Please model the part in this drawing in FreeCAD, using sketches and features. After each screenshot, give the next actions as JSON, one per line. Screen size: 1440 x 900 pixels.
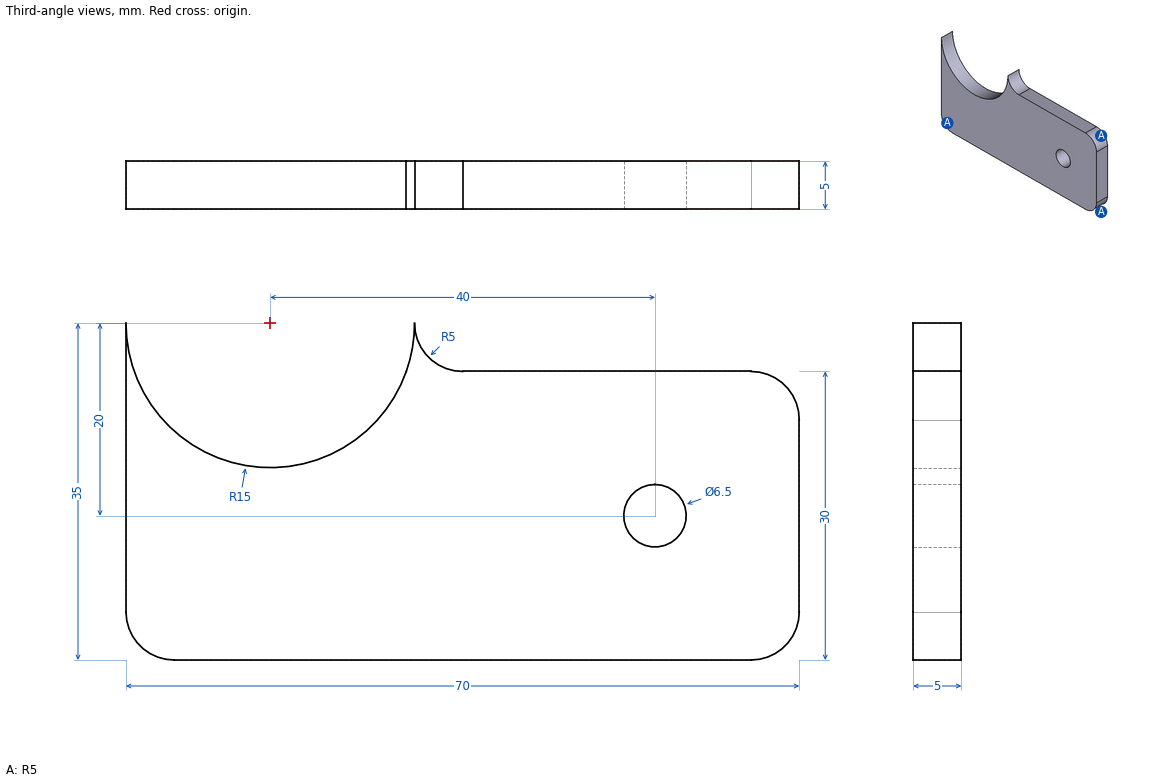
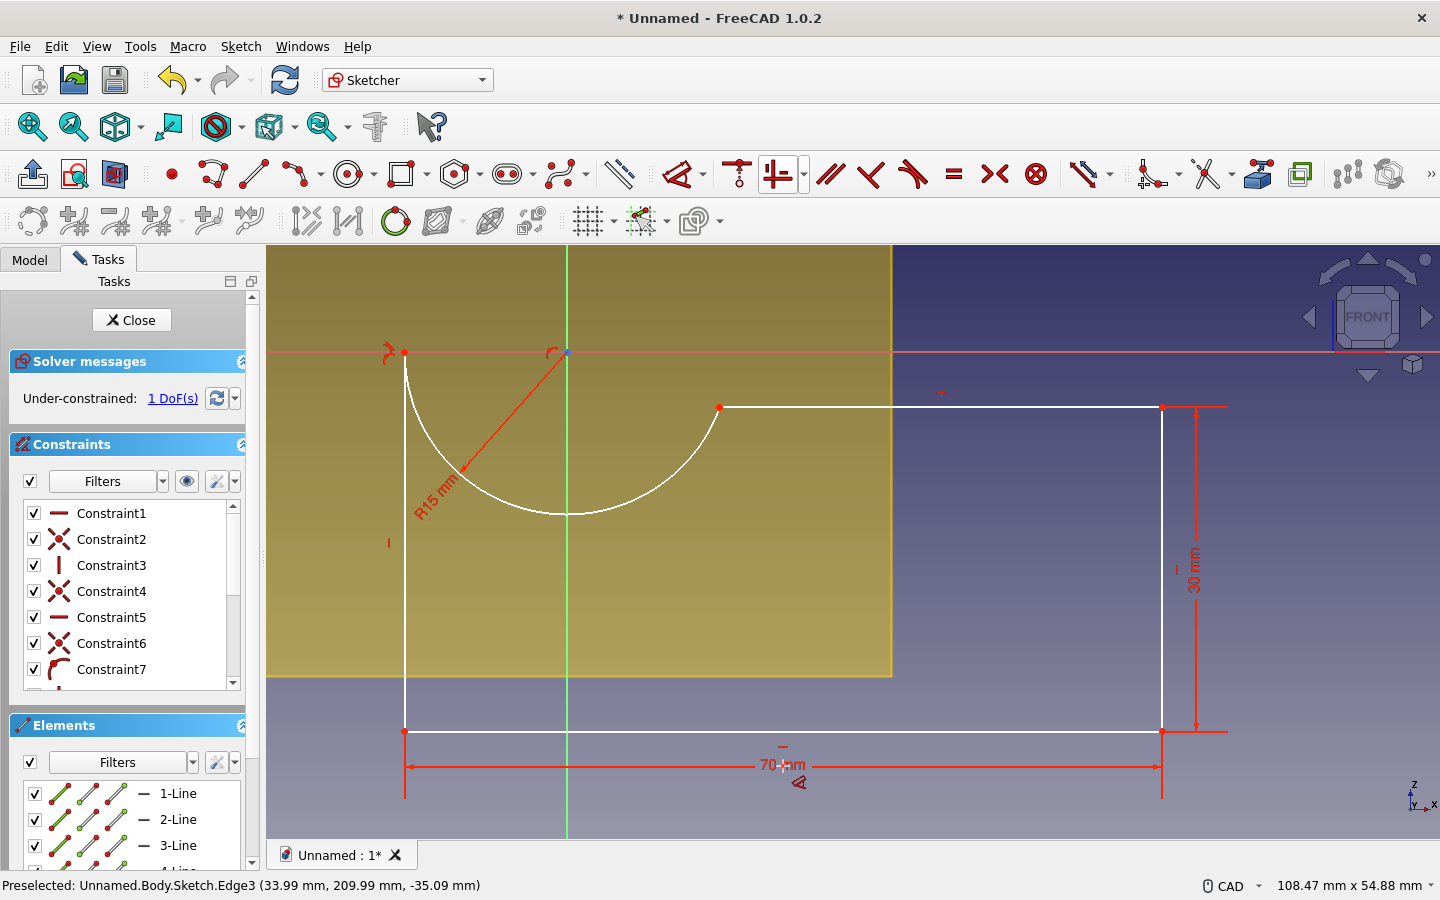
{"action": "left_click", "coordinate": [405, 618]}
{"action": "left_click", "coordinate": [371, 542]}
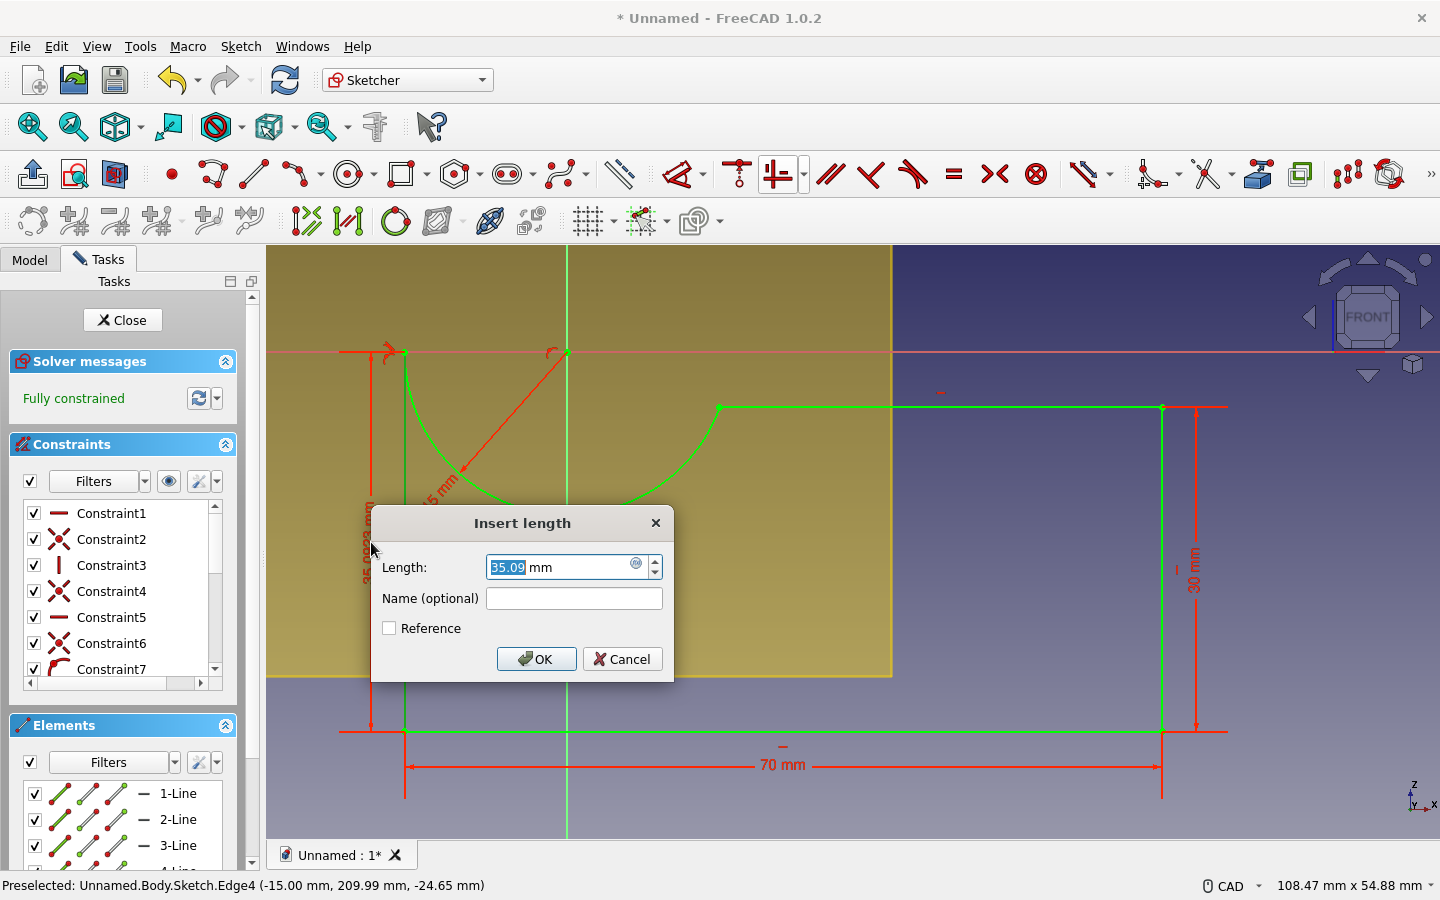
{"action": "type", "text": "35"}
{"action": "key", "text": "Return"}
{"action": "key", "text": "Escape"}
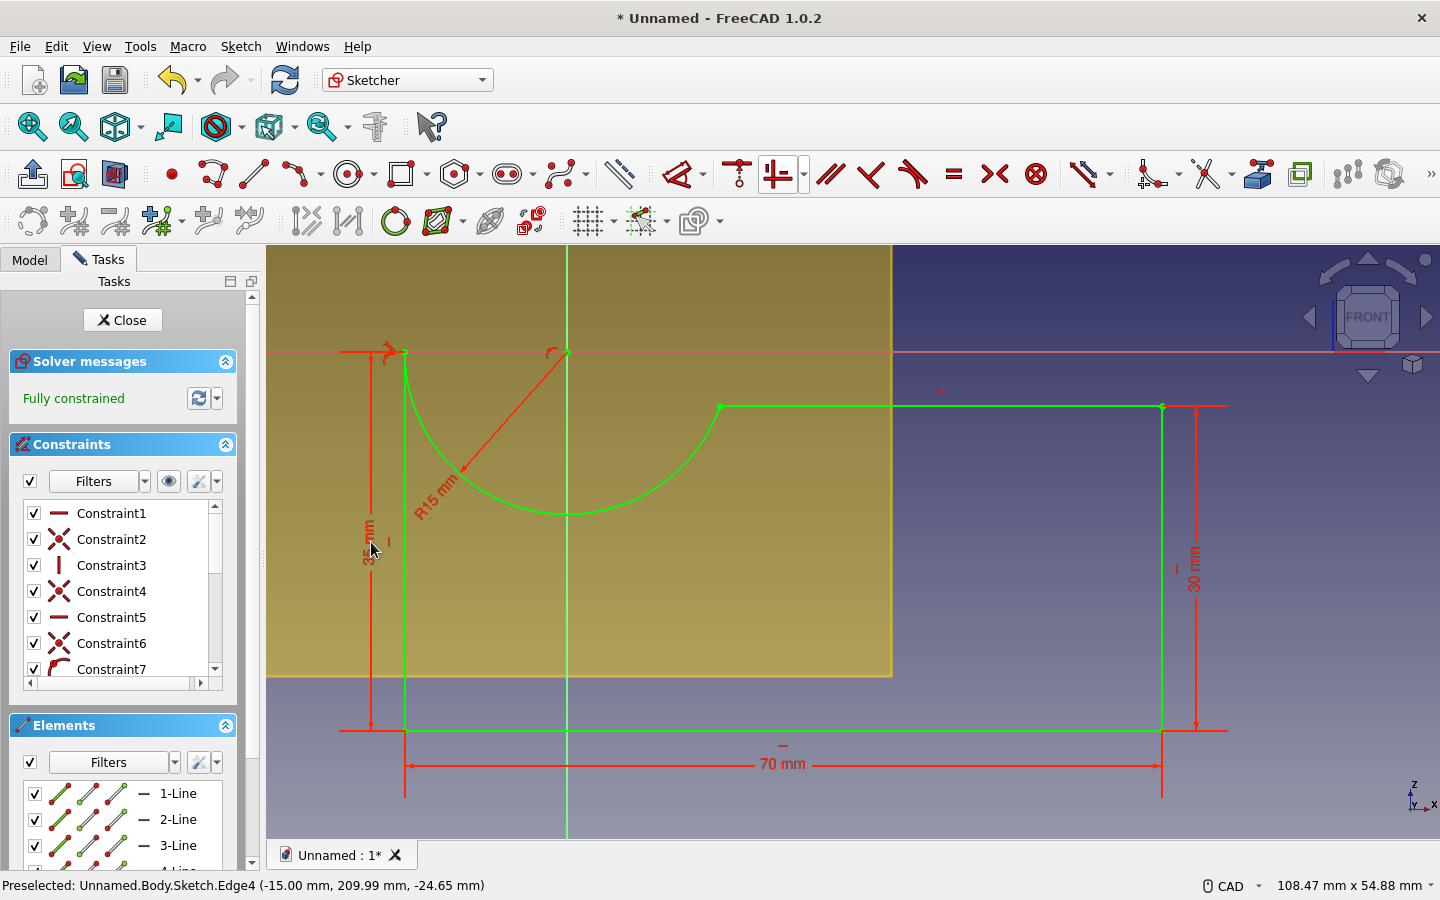
{"action": "left_click", "coordinate": [123, 320]}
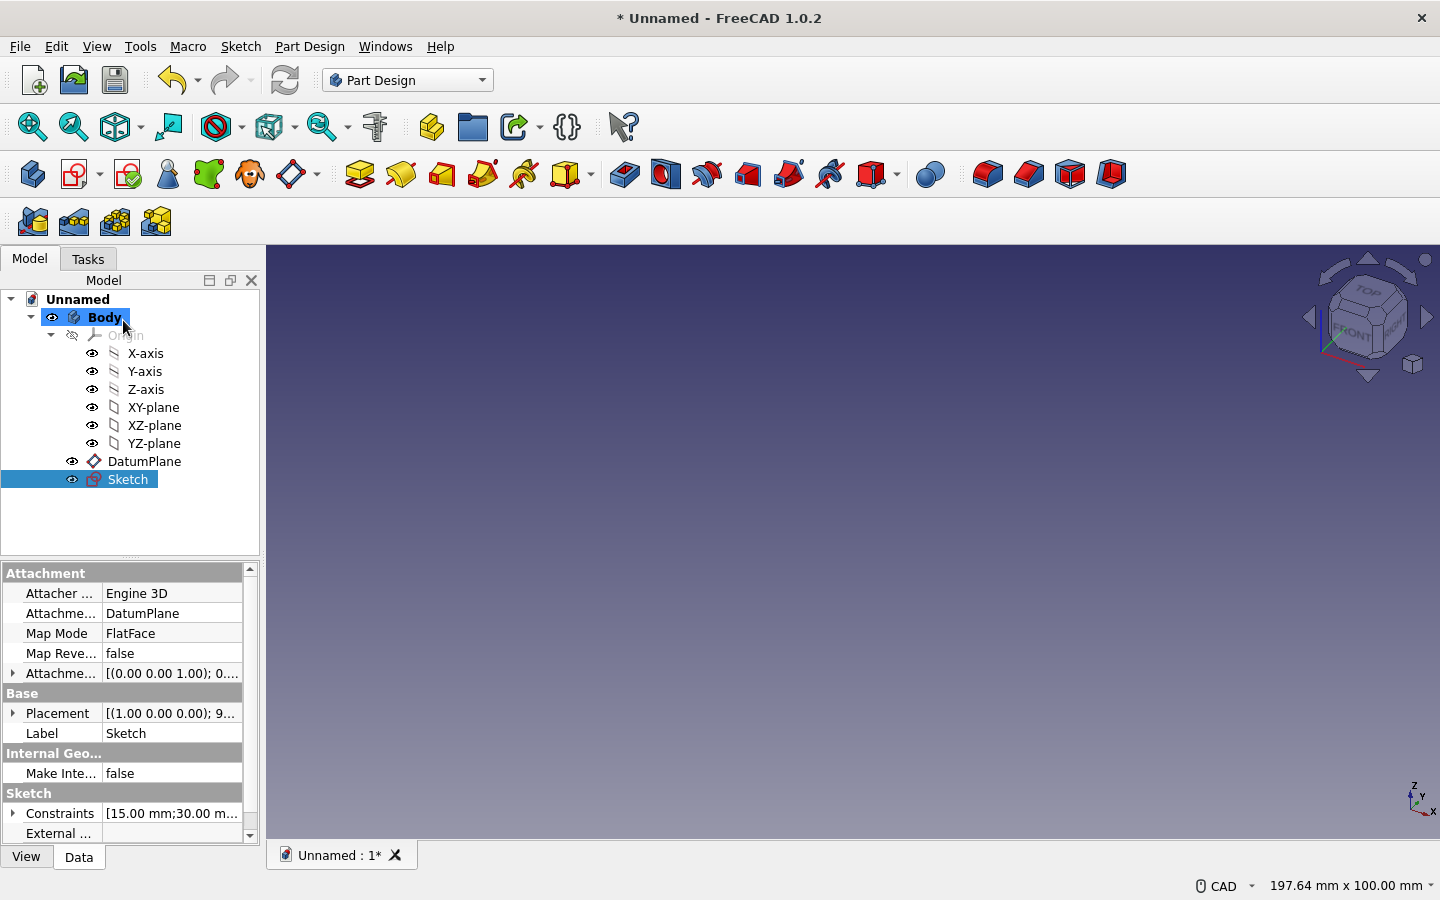
{"action": "left_click", "coordinate": [360, 174]}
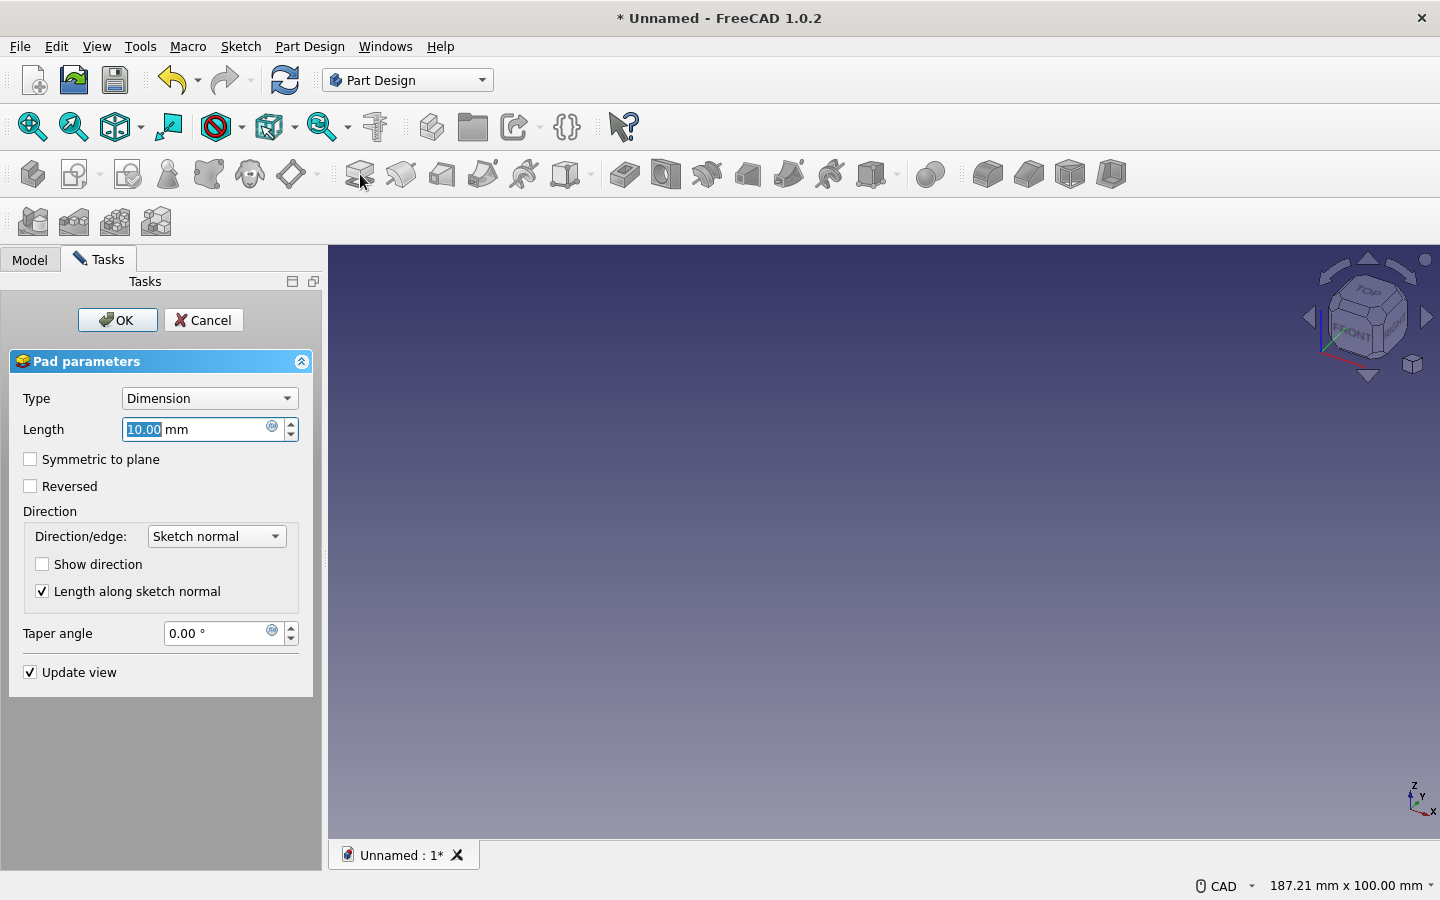
{"action": "type", "text": "5"}
{"action": "key", "text": "Tab"}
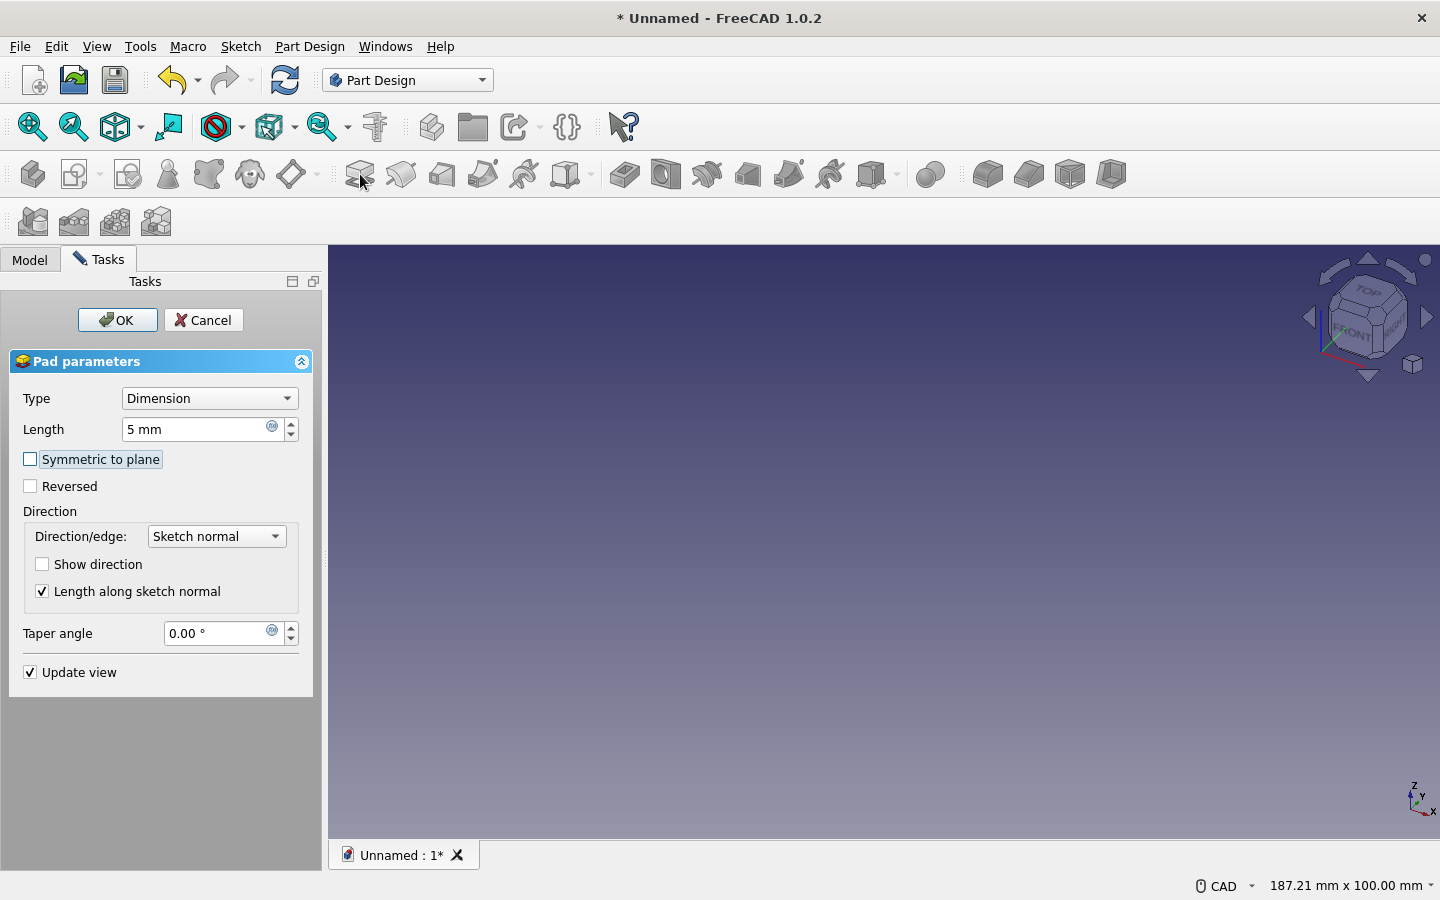
{"action": "left_click", "coordinate": [118, 320]}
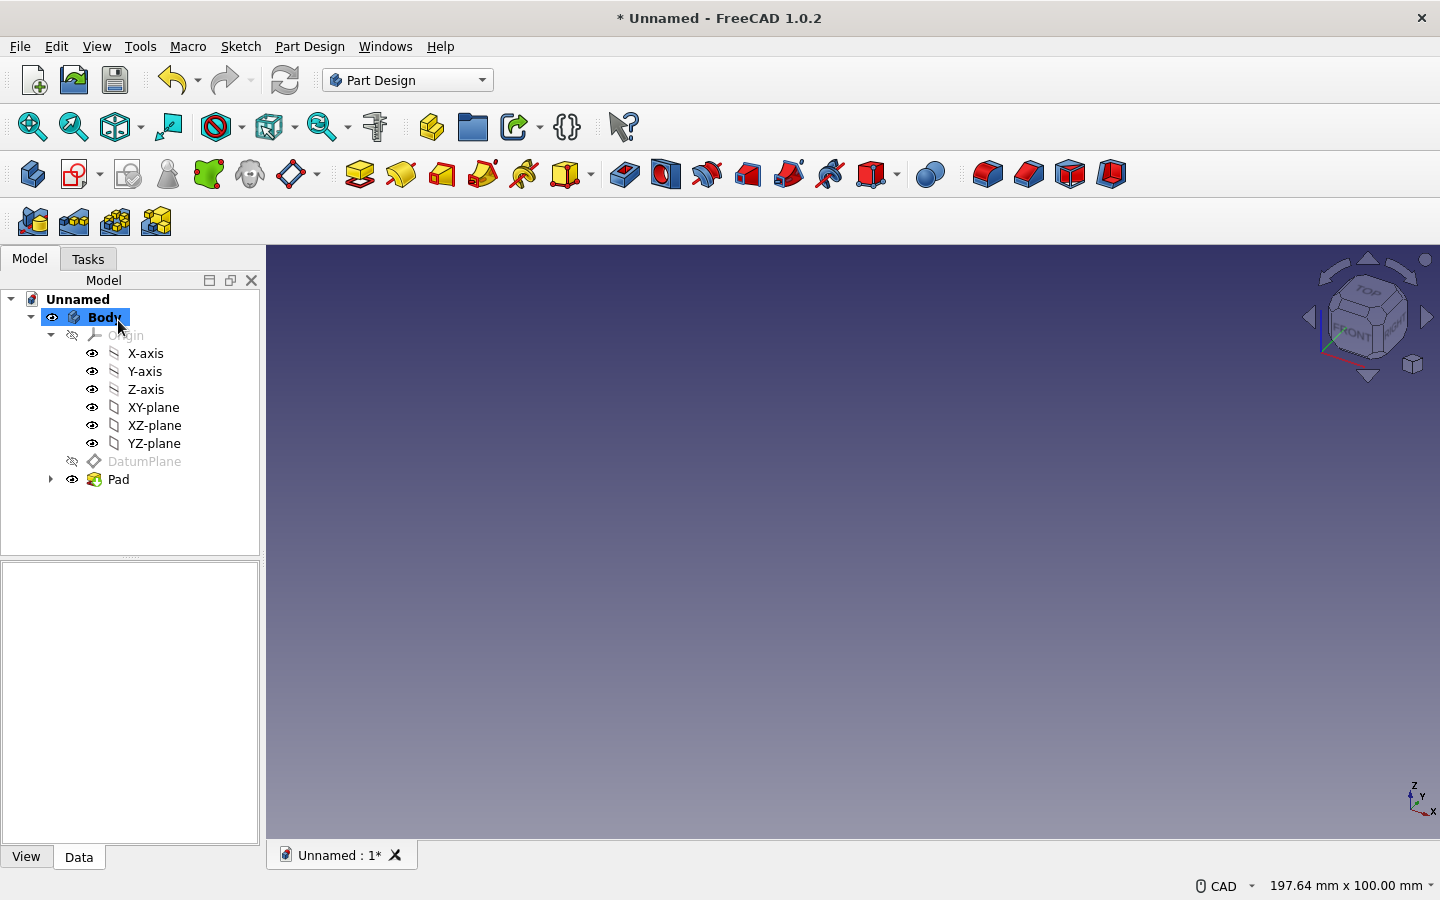
{"action": "left_click", "coordinate": [33, 128]}